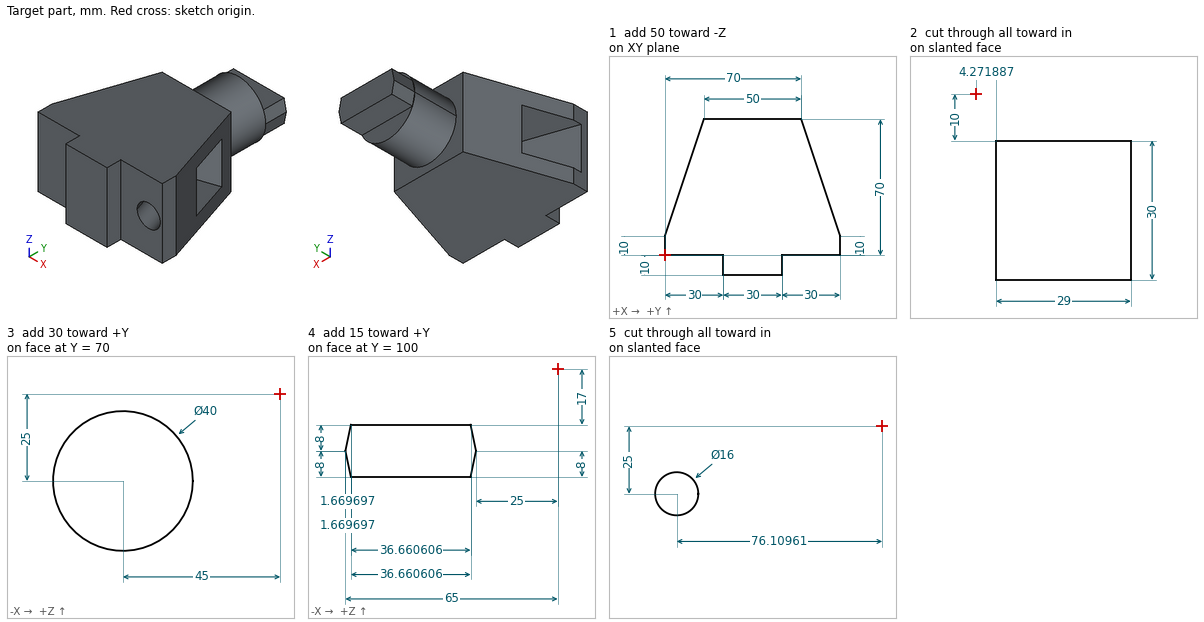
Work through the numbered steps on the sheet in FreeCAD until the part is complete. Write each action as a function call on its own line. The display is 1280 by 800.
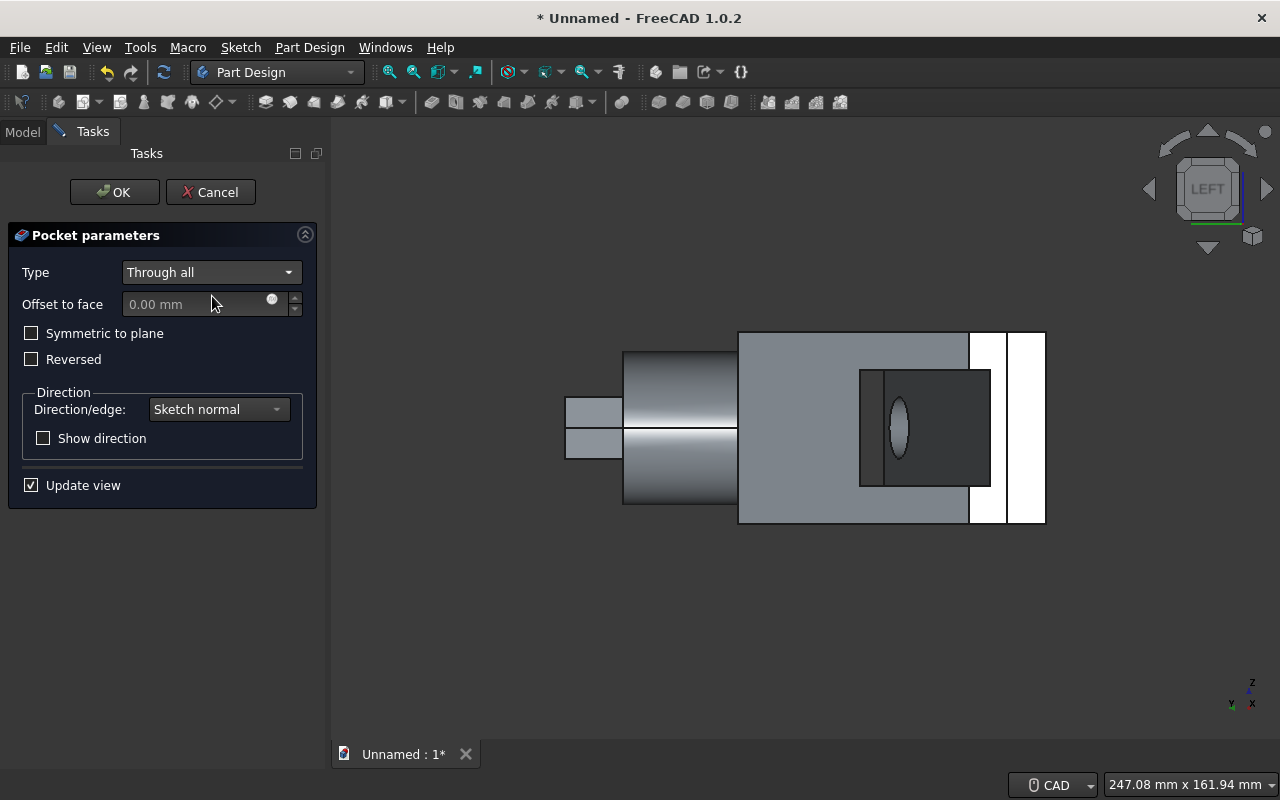
click(115, 192)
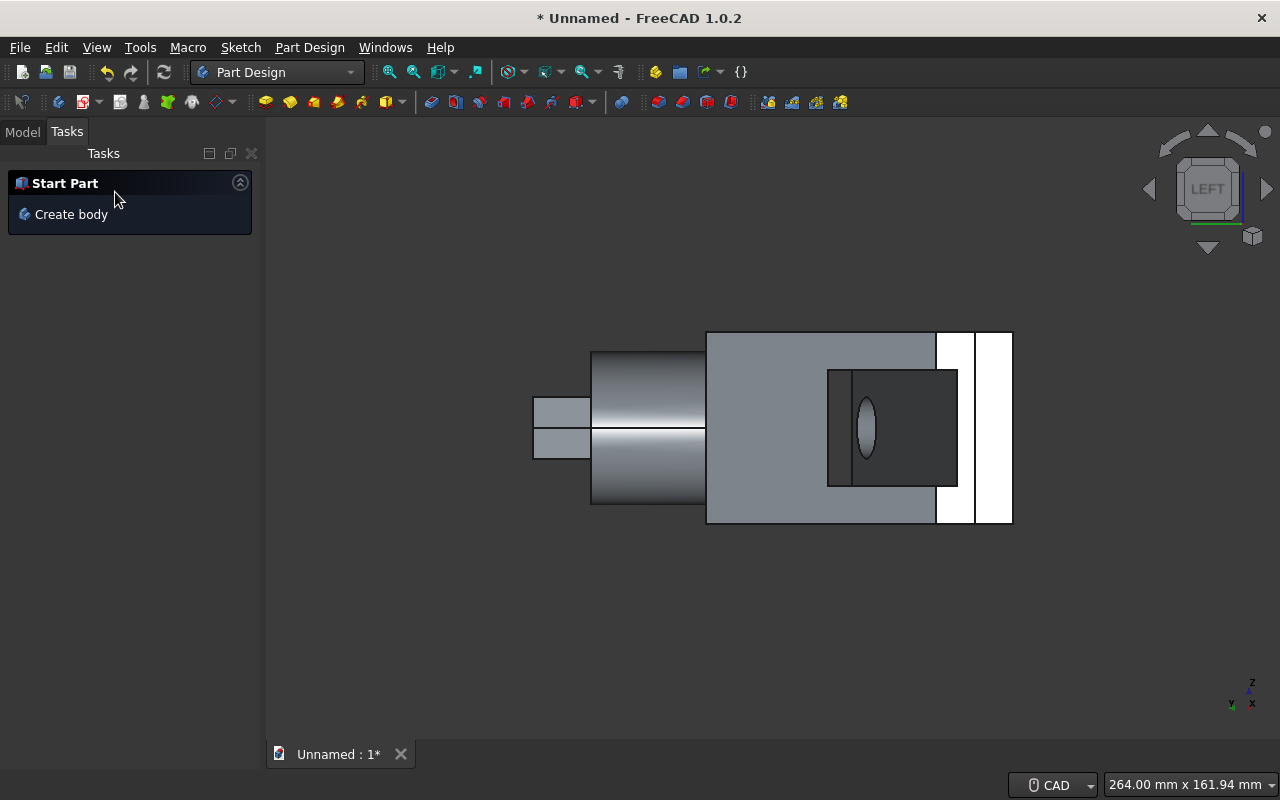
key(0)